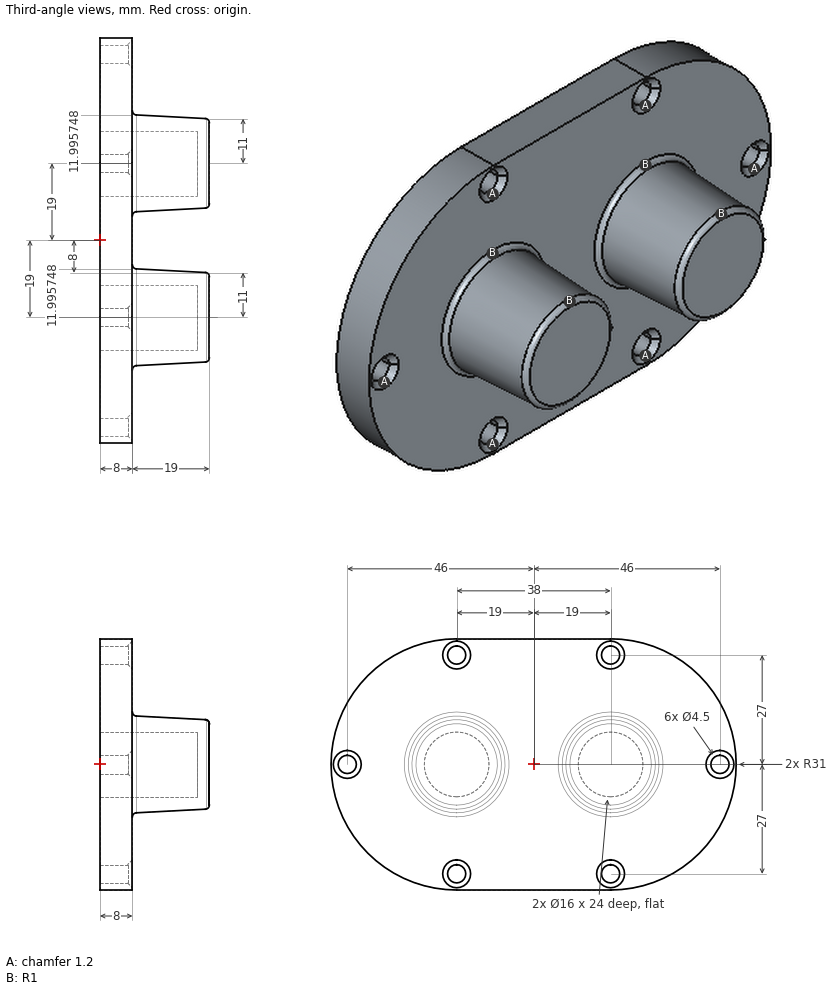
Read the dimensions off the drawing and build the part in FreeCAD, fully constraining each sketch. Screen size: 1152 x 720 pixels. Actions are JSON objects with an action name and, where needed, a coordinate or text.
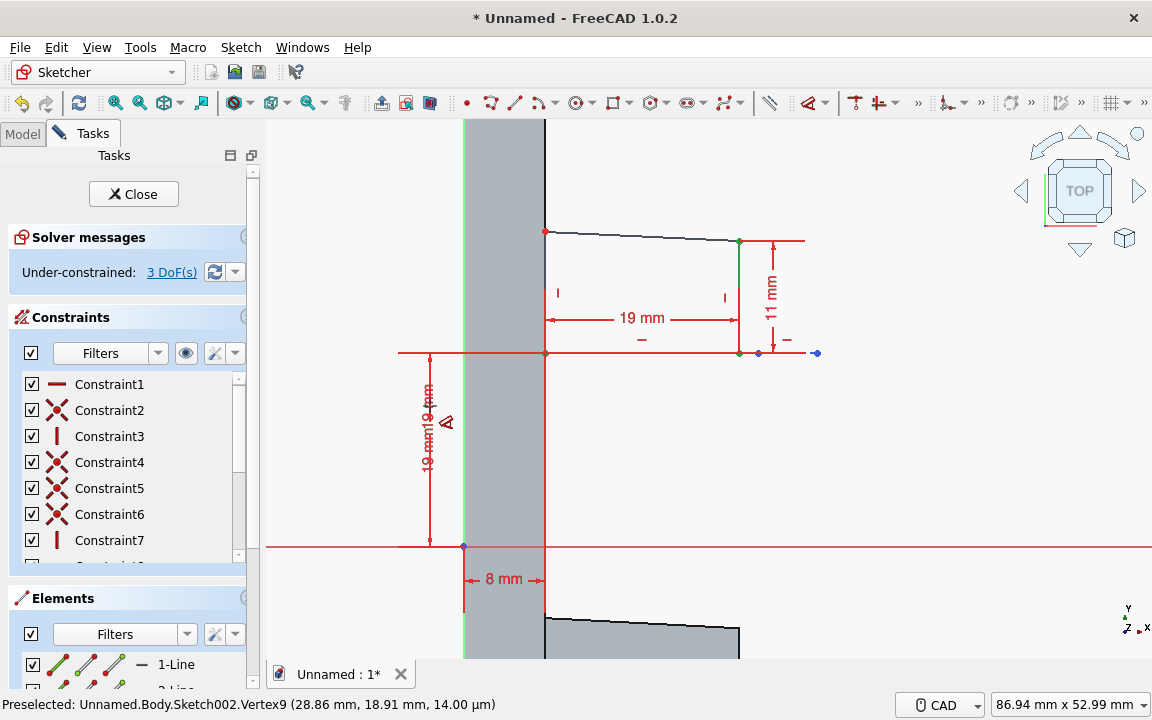
{"action": "left_click", "coordinate": [545, 268]}
{"action": "left_click", "coordinate": [511, 293]}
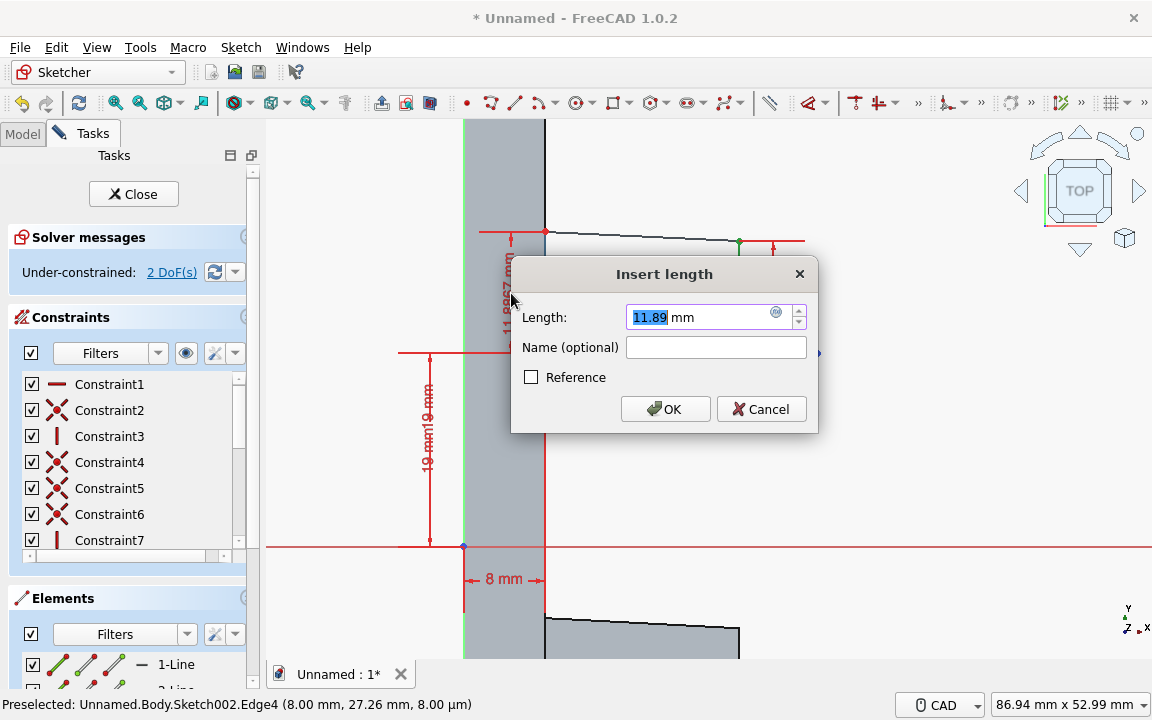
{"action": "type", "text": "11.995748"}
{"action": "key", "text": "Return"}
{"action": "key", "text": "Escape"}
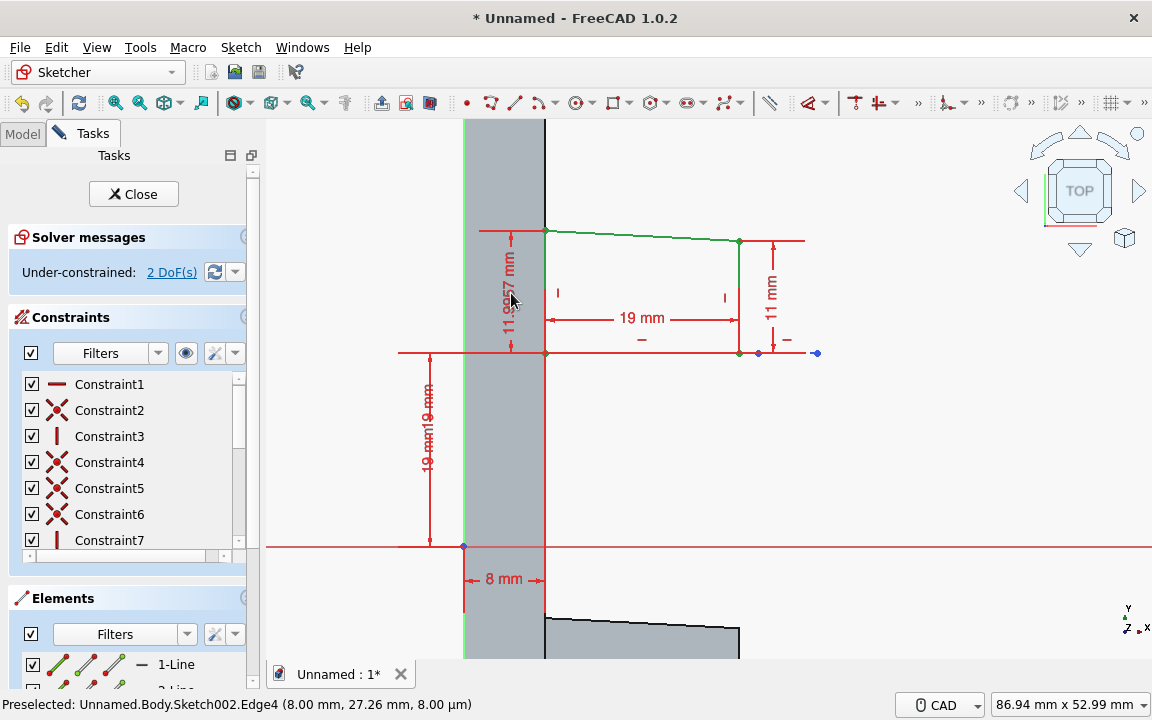
{"action": "left_click", "coordinate": [134, 194]}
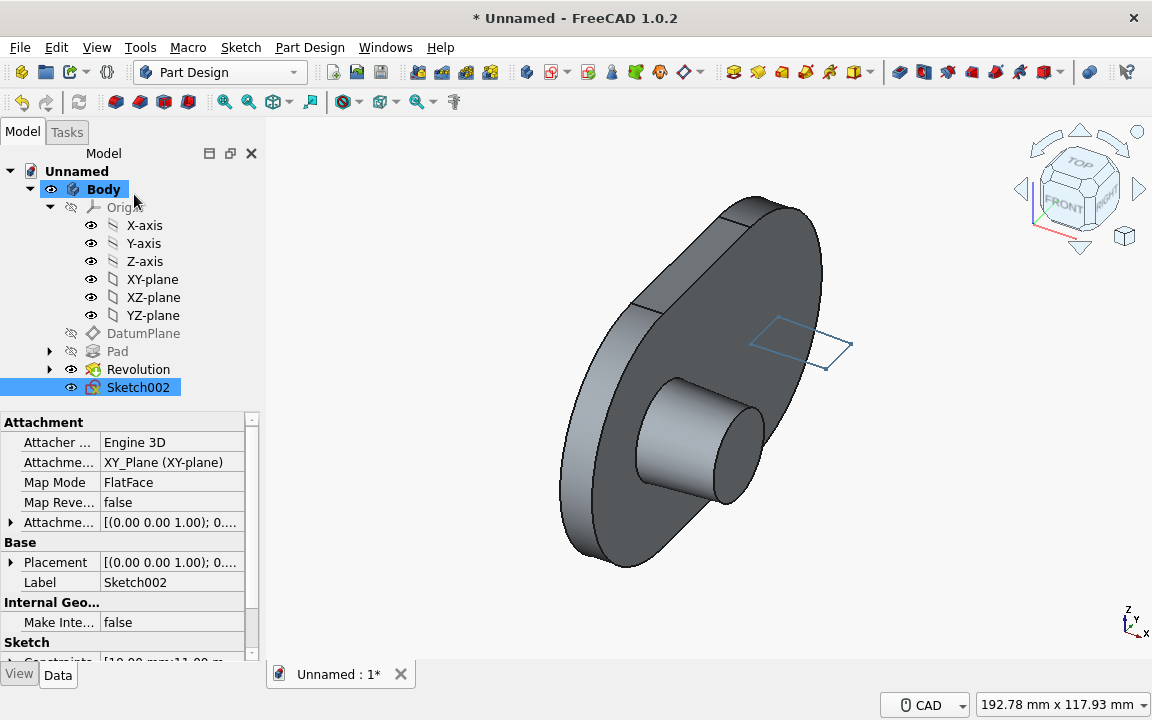
{"action": "left_click", "coordinate": [758, 72]}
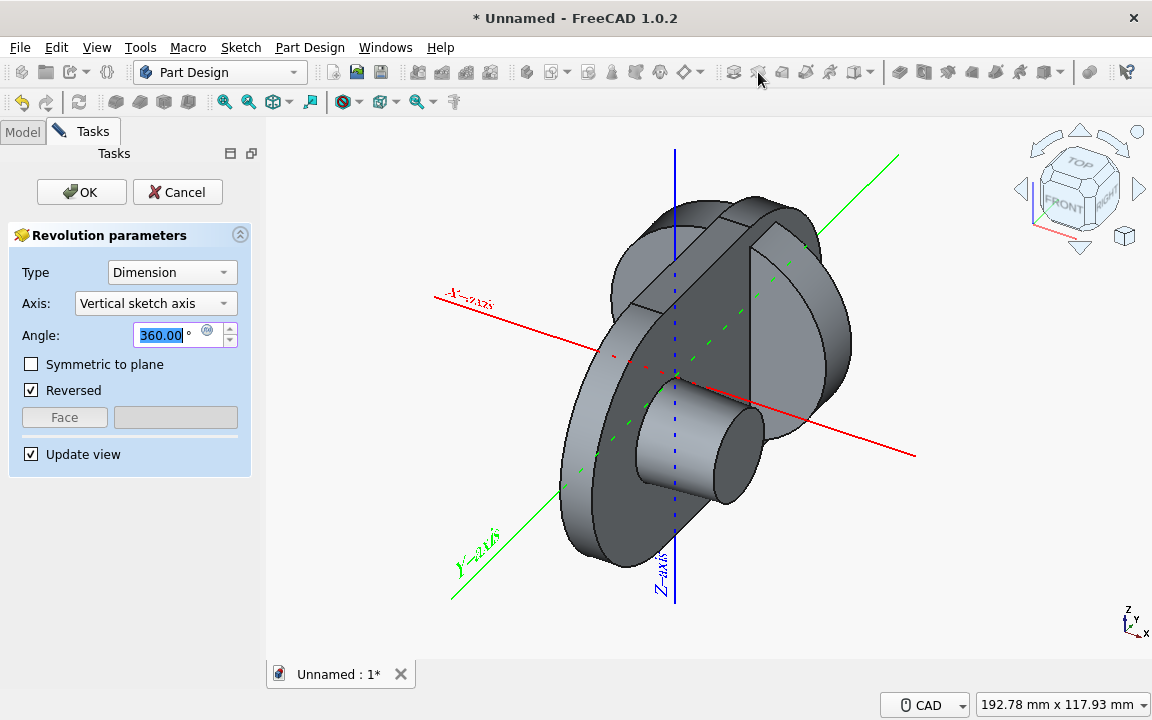
{"action": "left_click", "coordinate": [156, 304]}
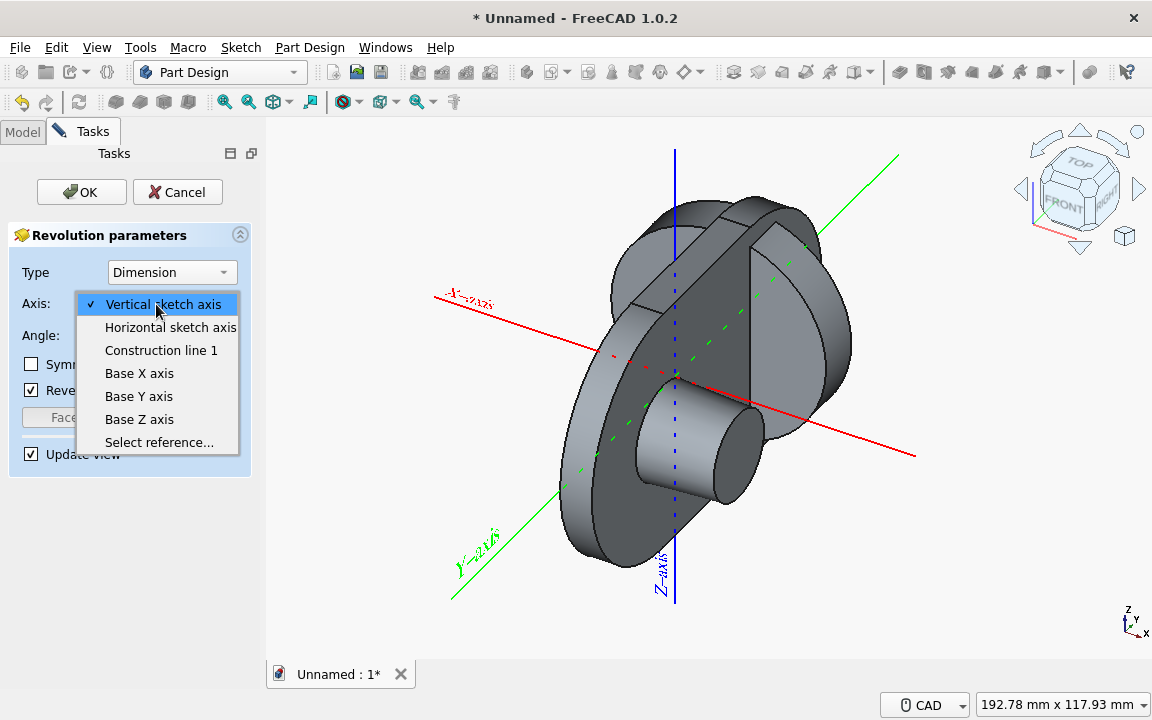
{"action": "left_click", "coordinate": [156, 350]}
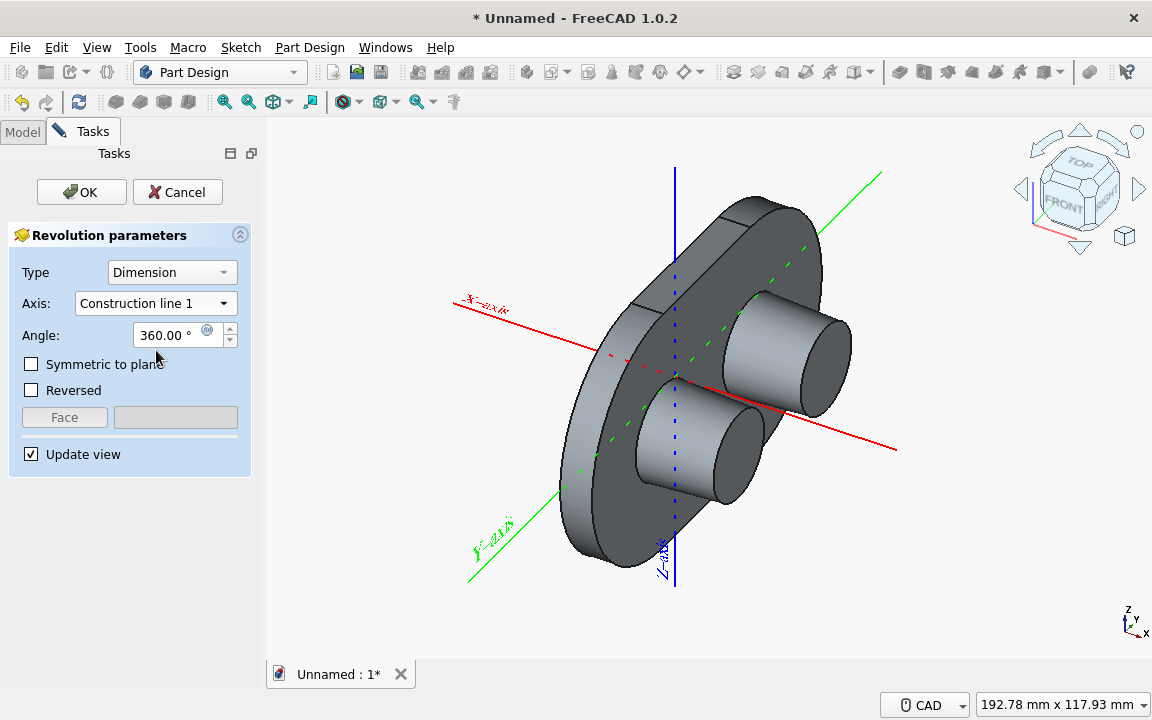
{"action": "left_click", "coordinate": [82, 192]}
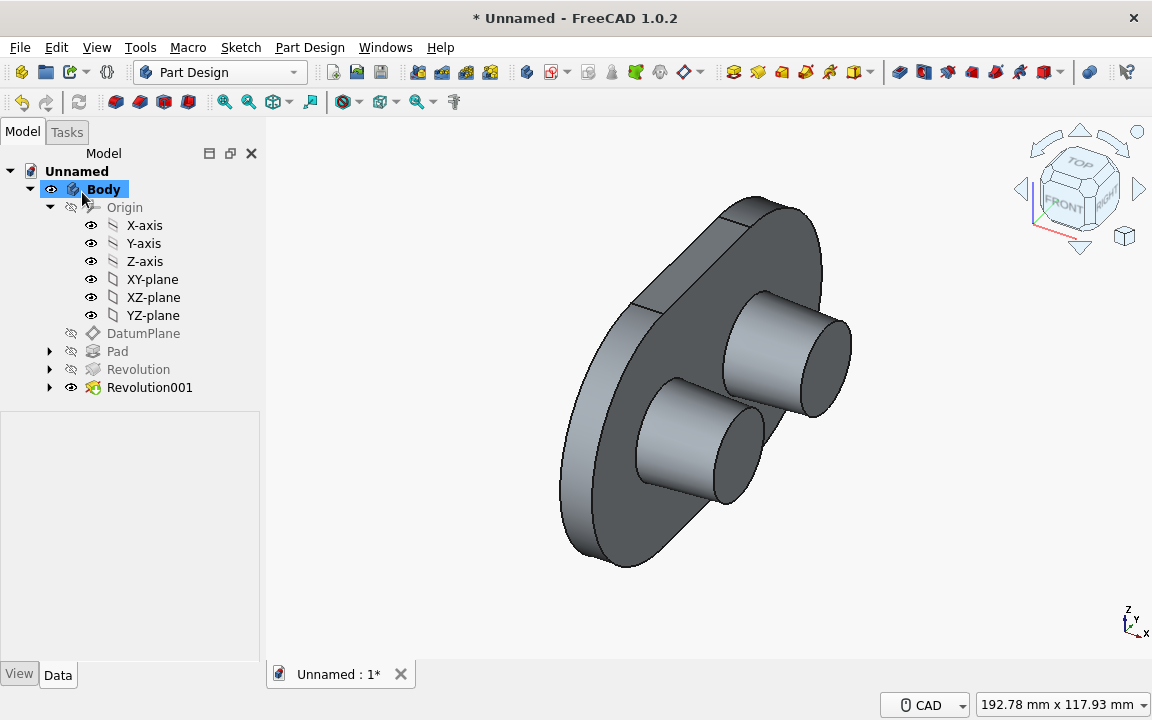
{"action": "left_click", "coordinate": [552, 72]}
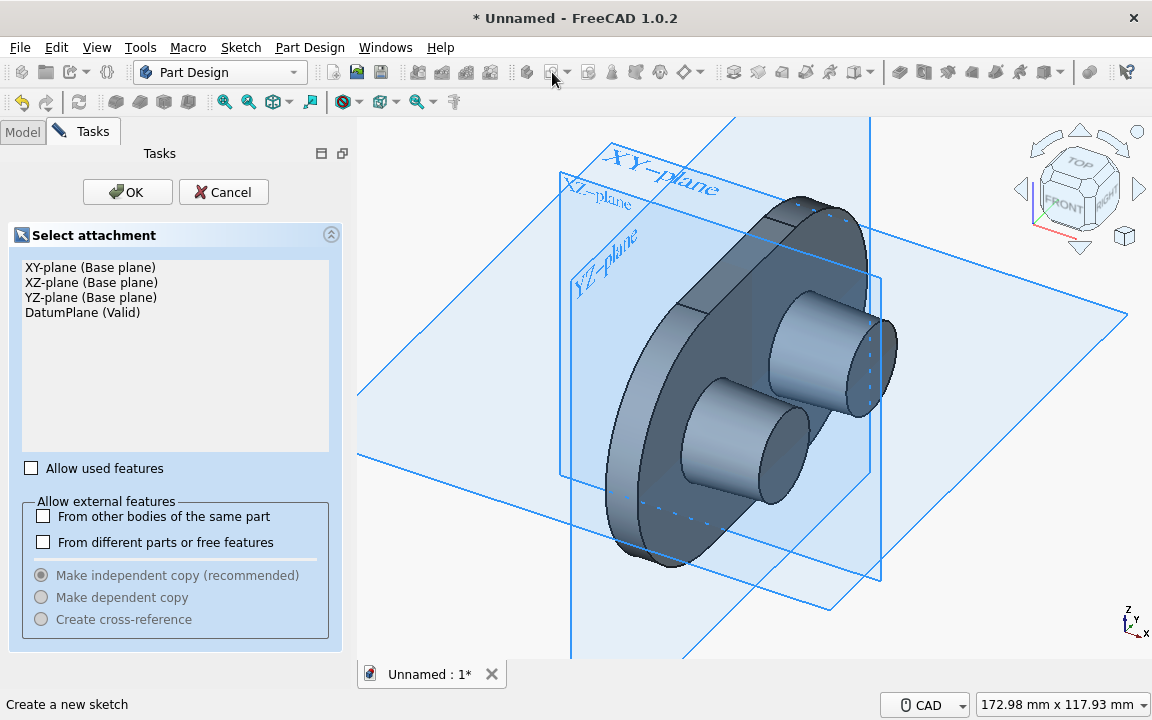
{"action": "left_click", "coordinate": [82, 298]}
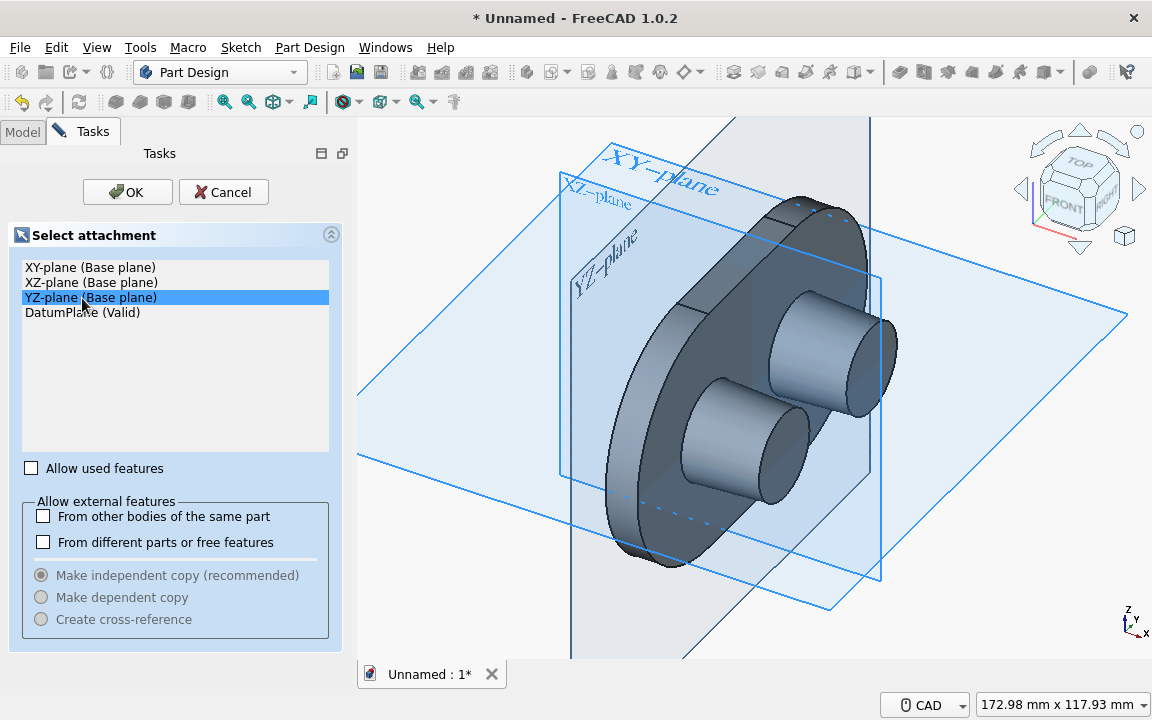
{"action": "left_click", "coordinate": [128, 192]}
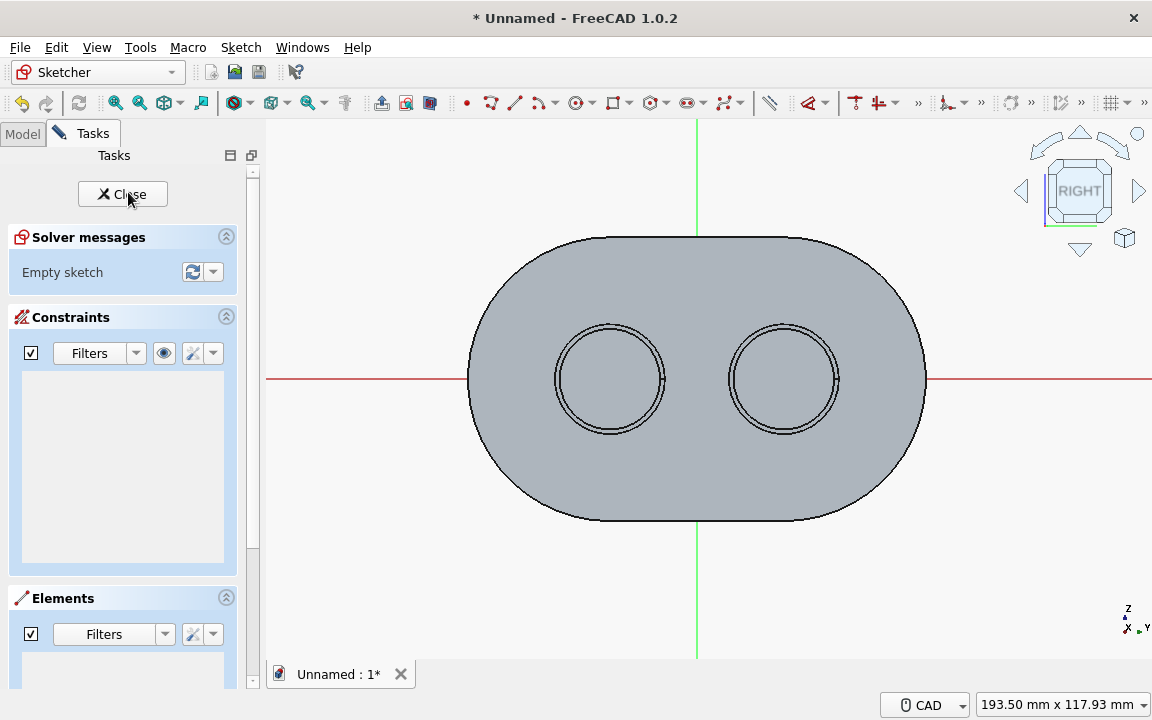
{"action": "left_click", "coordinate": [430, 104]}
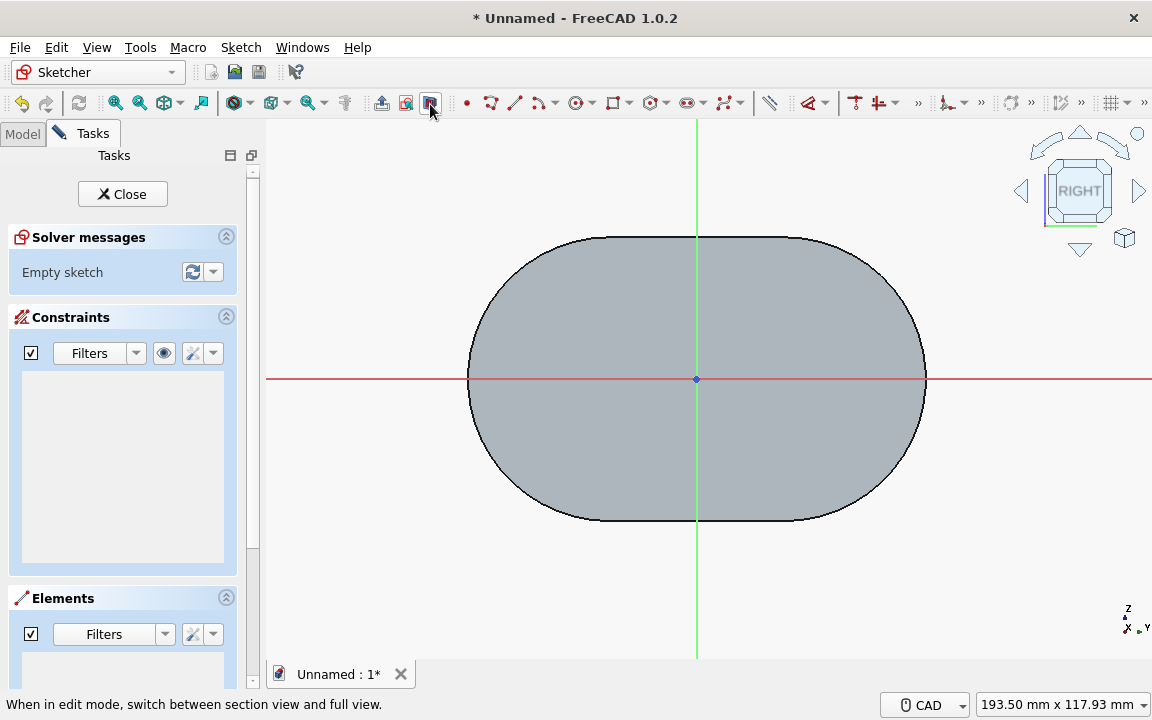
{"action": "scroll", "coordinate": [765, 367], "scroll_direction": "up", "scroll_amount": 3}